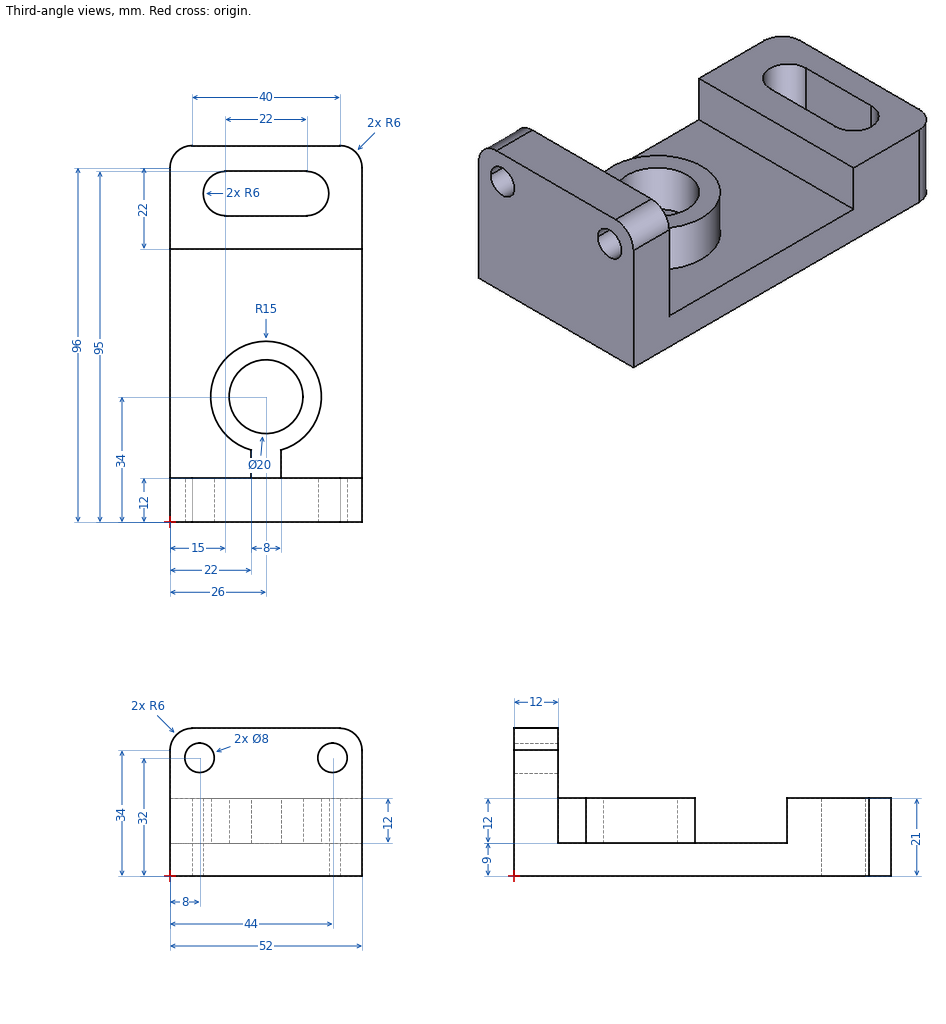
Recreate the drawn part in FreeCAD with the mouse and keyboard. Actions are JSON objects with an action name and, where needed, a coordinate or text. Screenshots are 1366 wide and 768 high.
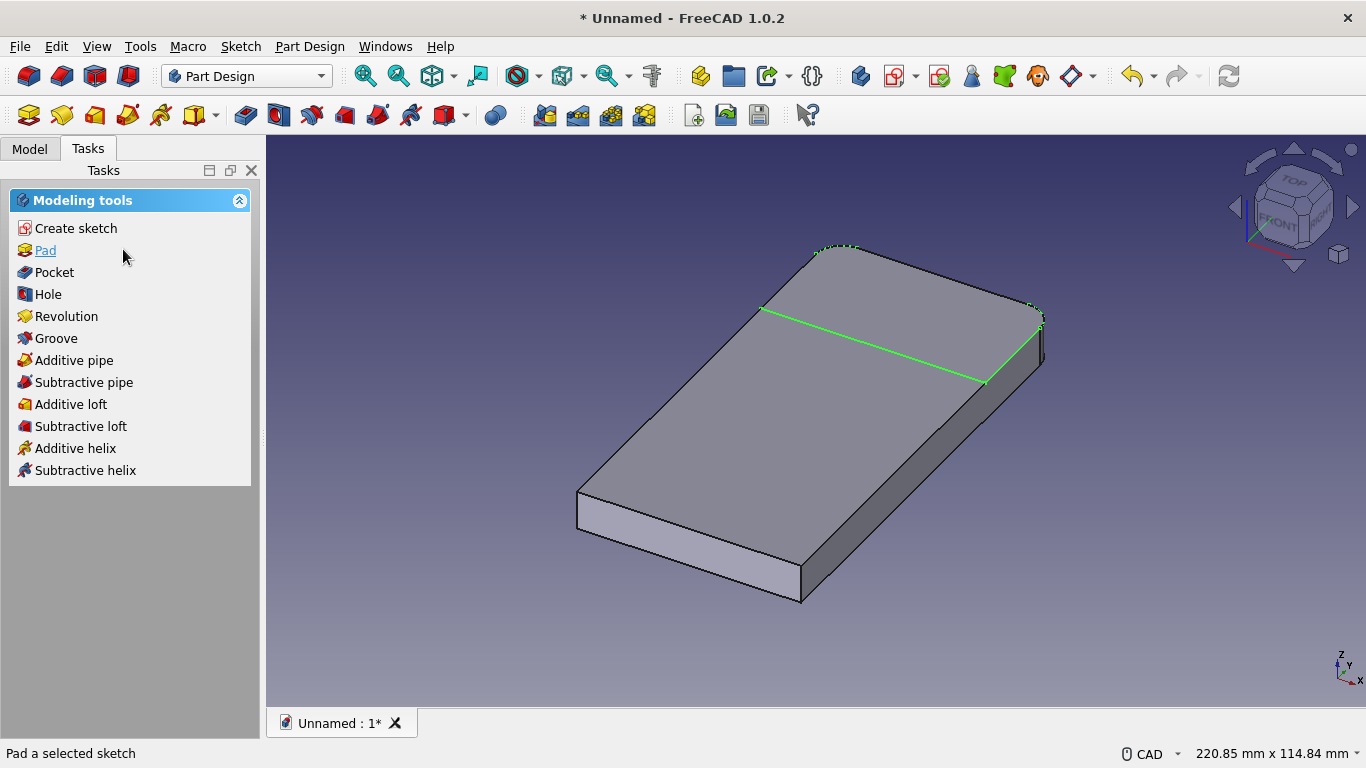
{"action": "left_click", "coordinate": [29, 116]}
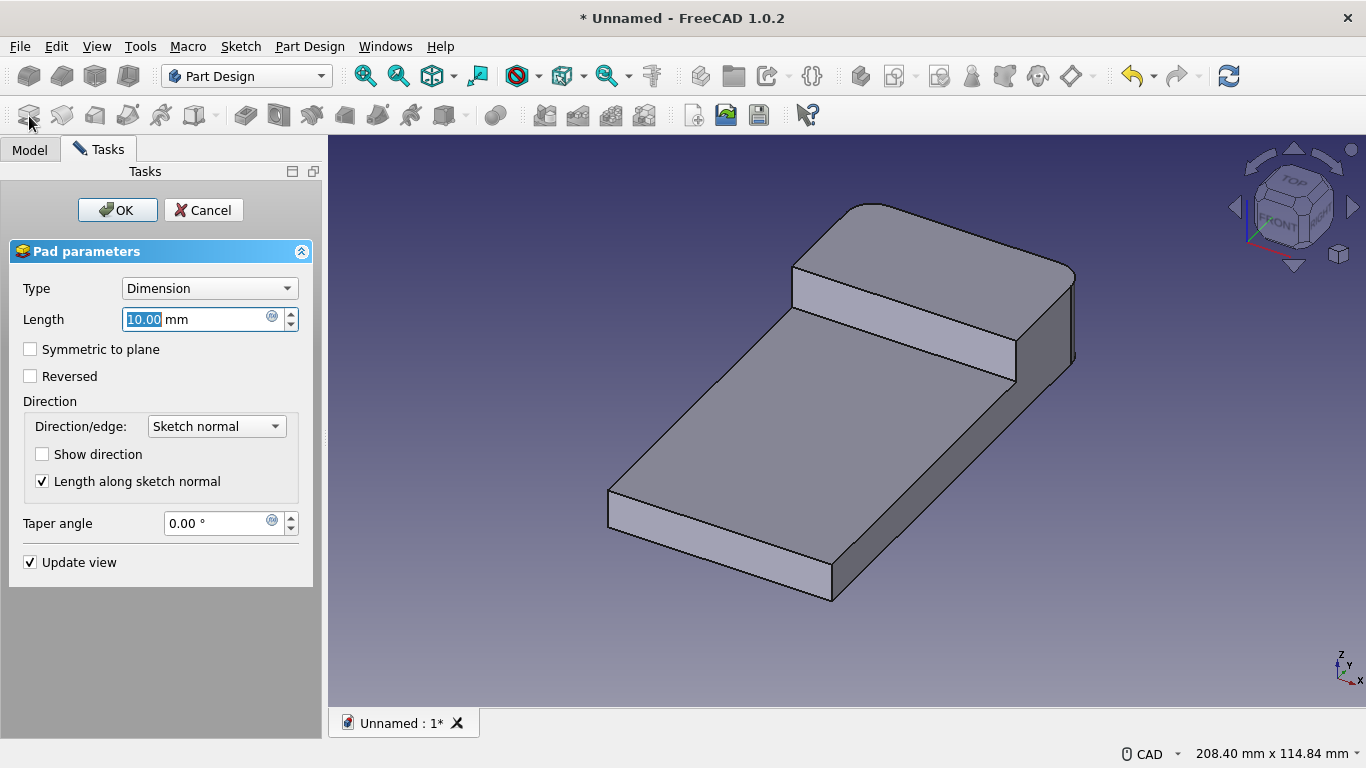
{"action": "type", "text": "12"}
{"action": "key", "text": "Tab"}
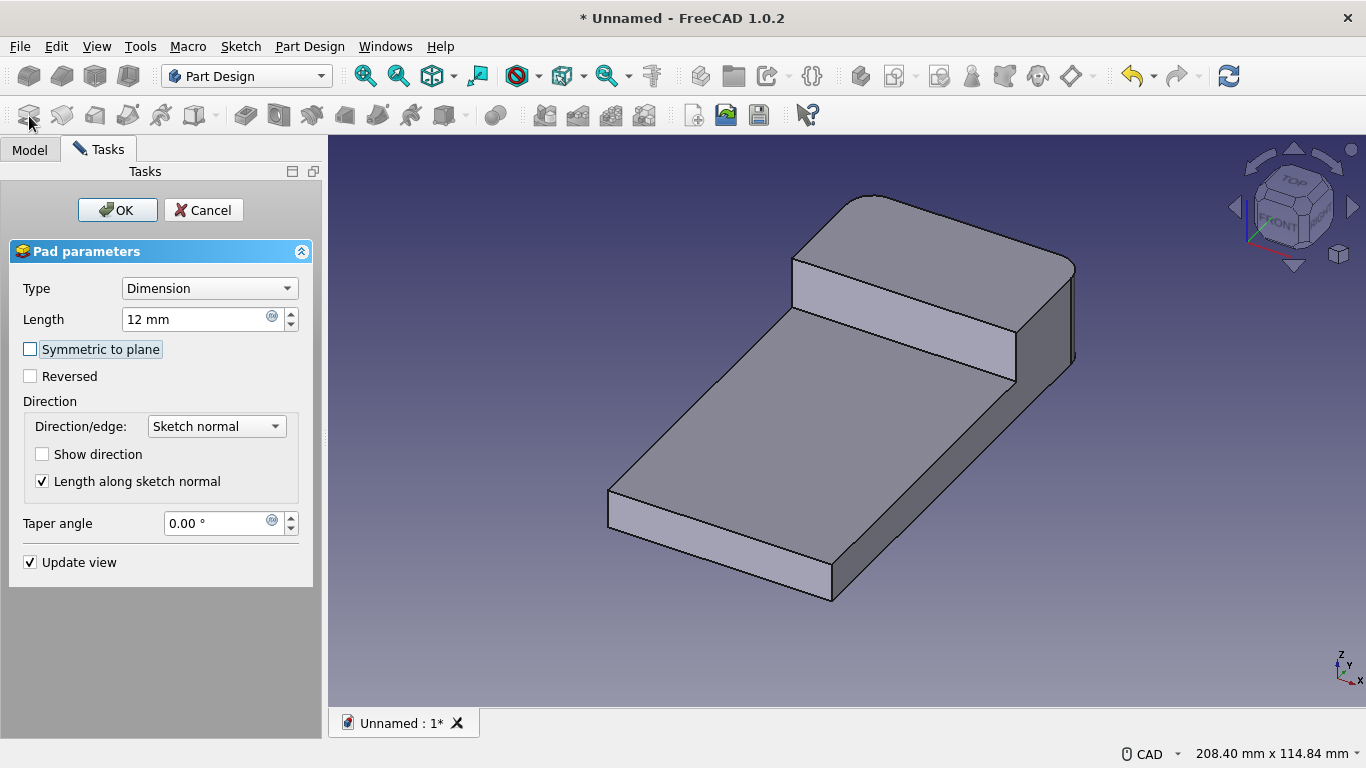
{"action": "left_click", "coordinate": [118, 210]}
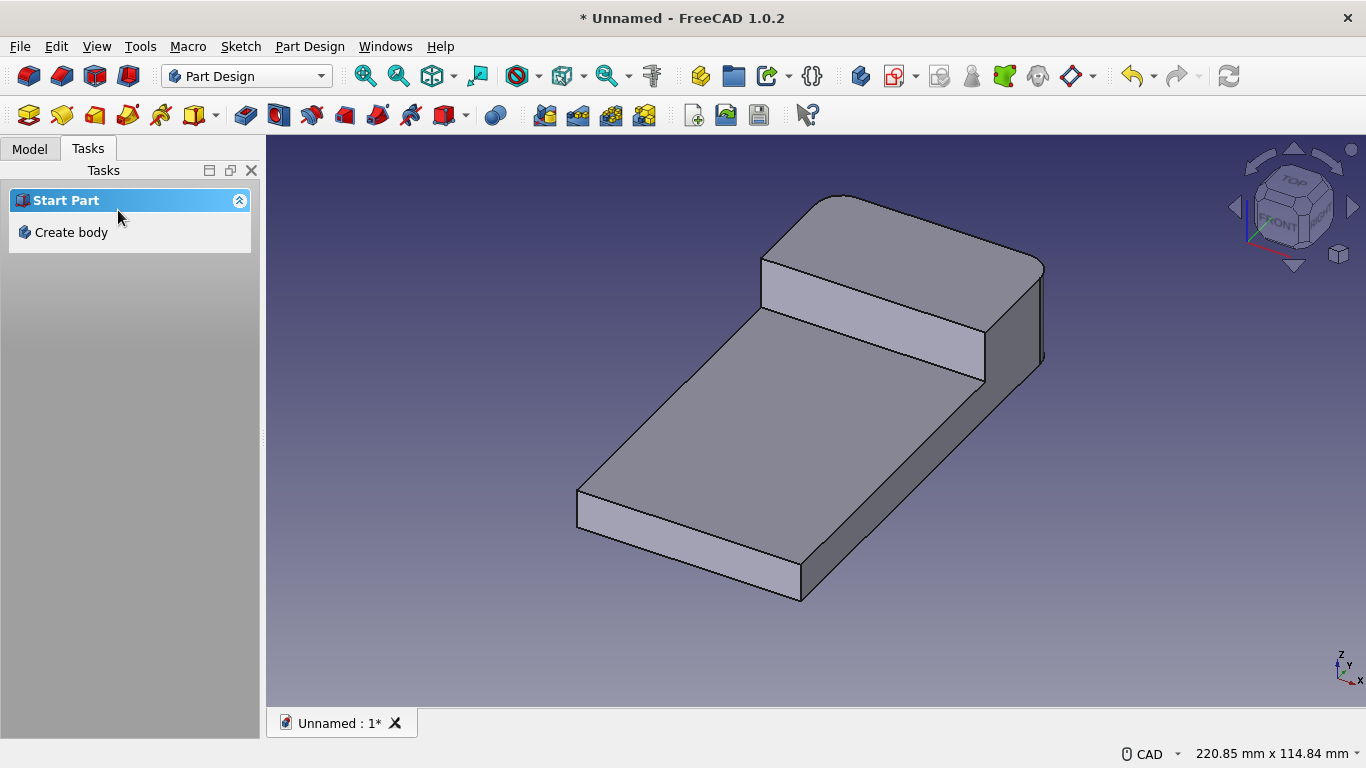
{"action": "left_click", "coordinate": [940, 271]}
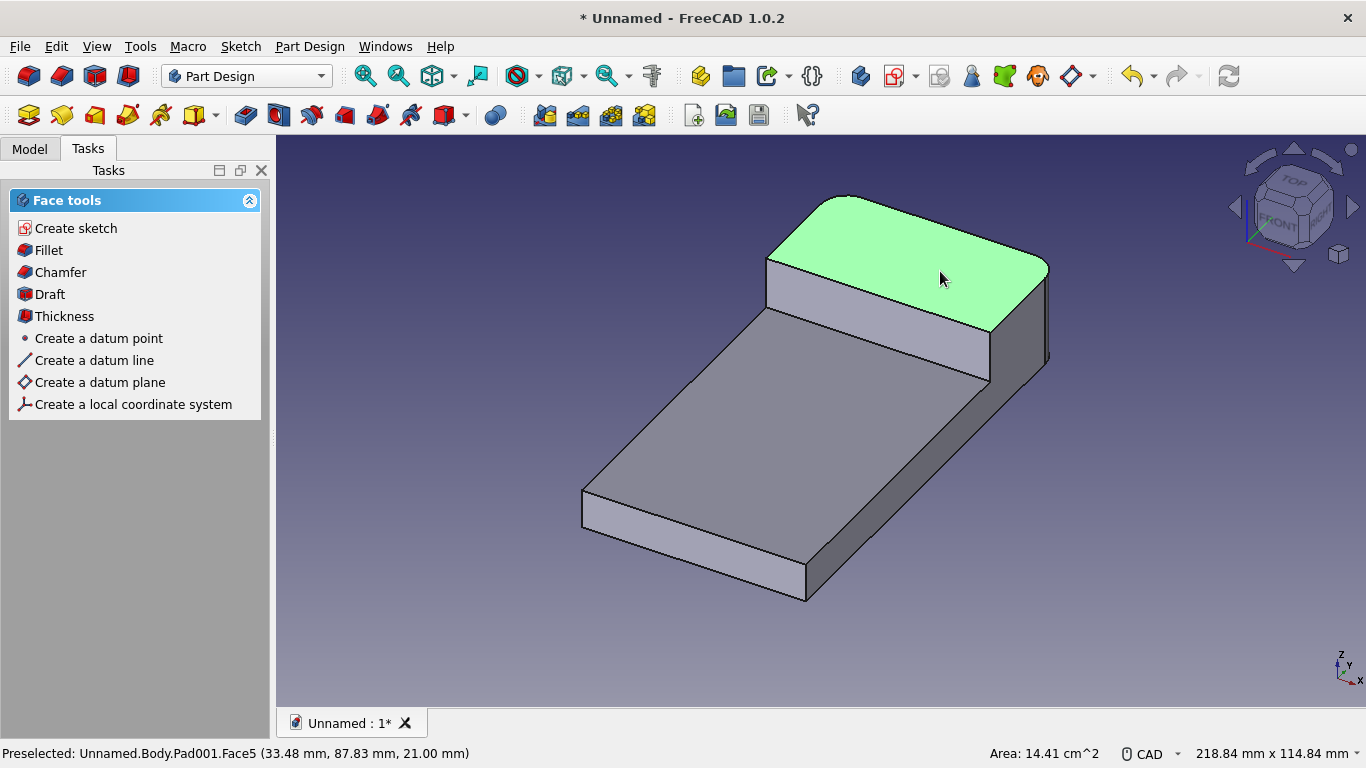
{"action": "left_click", "coordinate": [894, 76]}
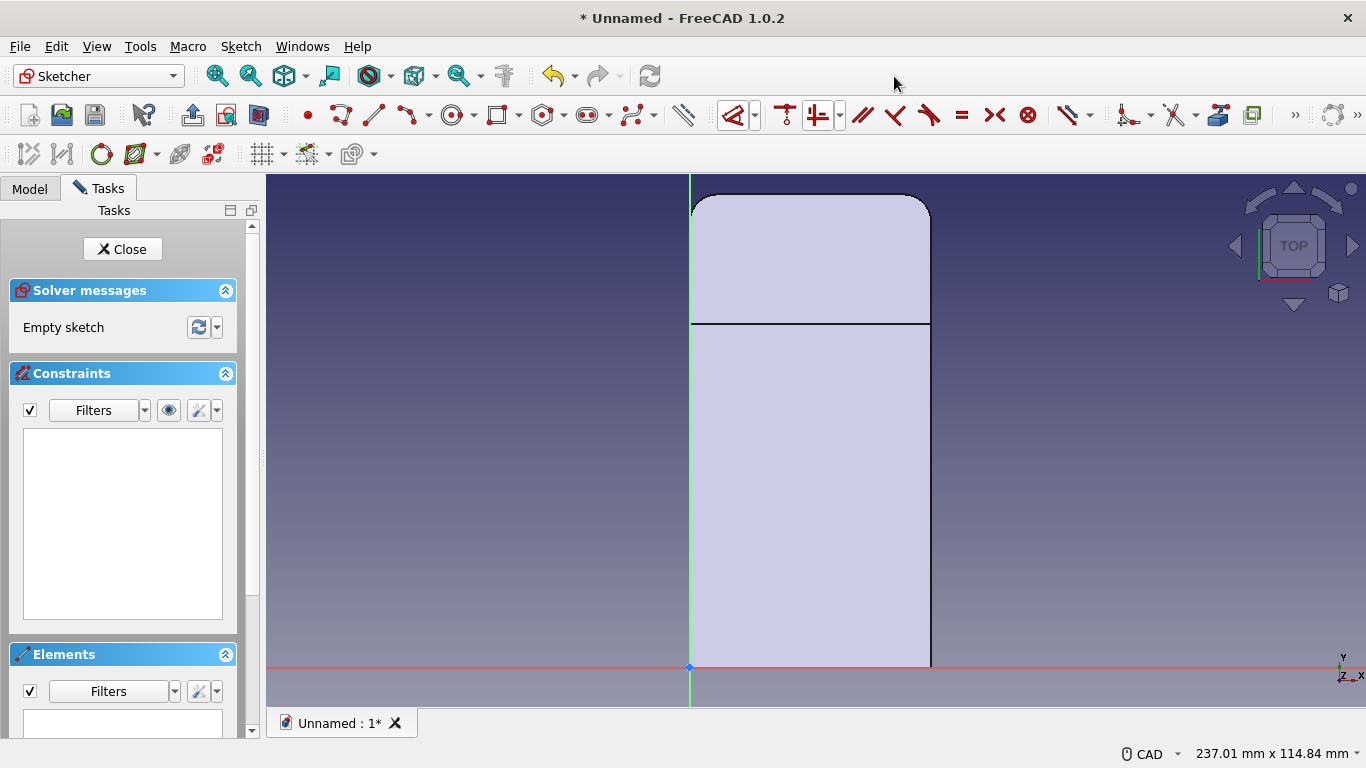
{"action": "scroll", "coordinate": [831, 202], "scroll_direction": "up", "scroll_amount": 7}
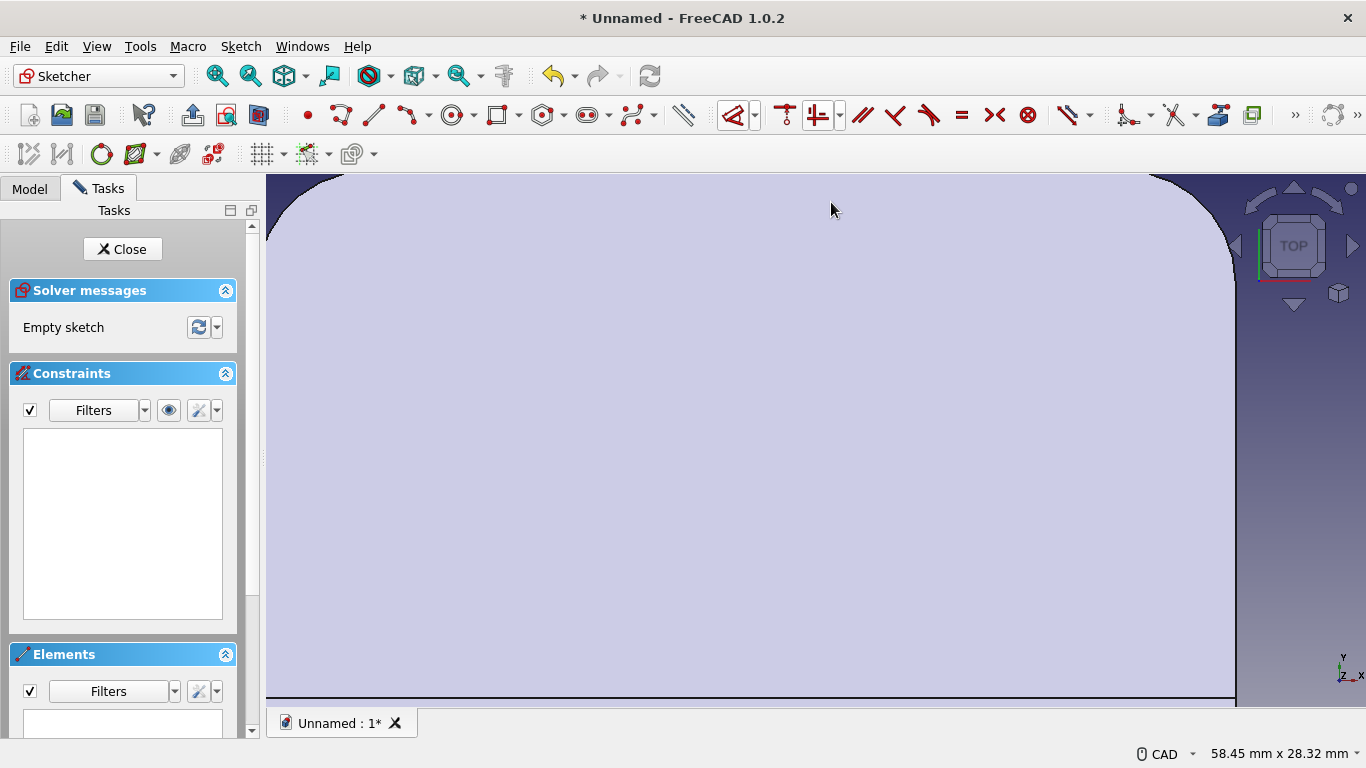
{"action": "left_click", "coordinate": [586, 116]}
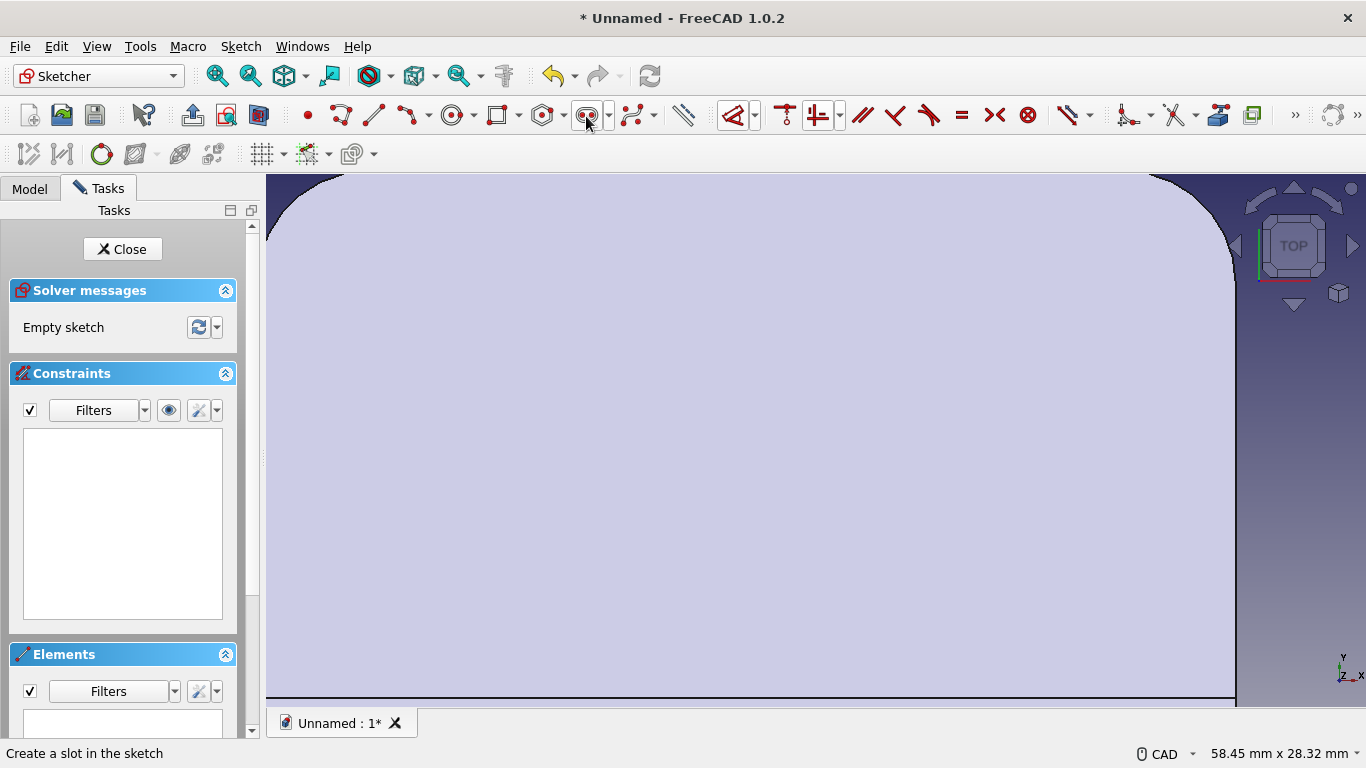
{"action": "left_click", "coordinate": [539, 415]}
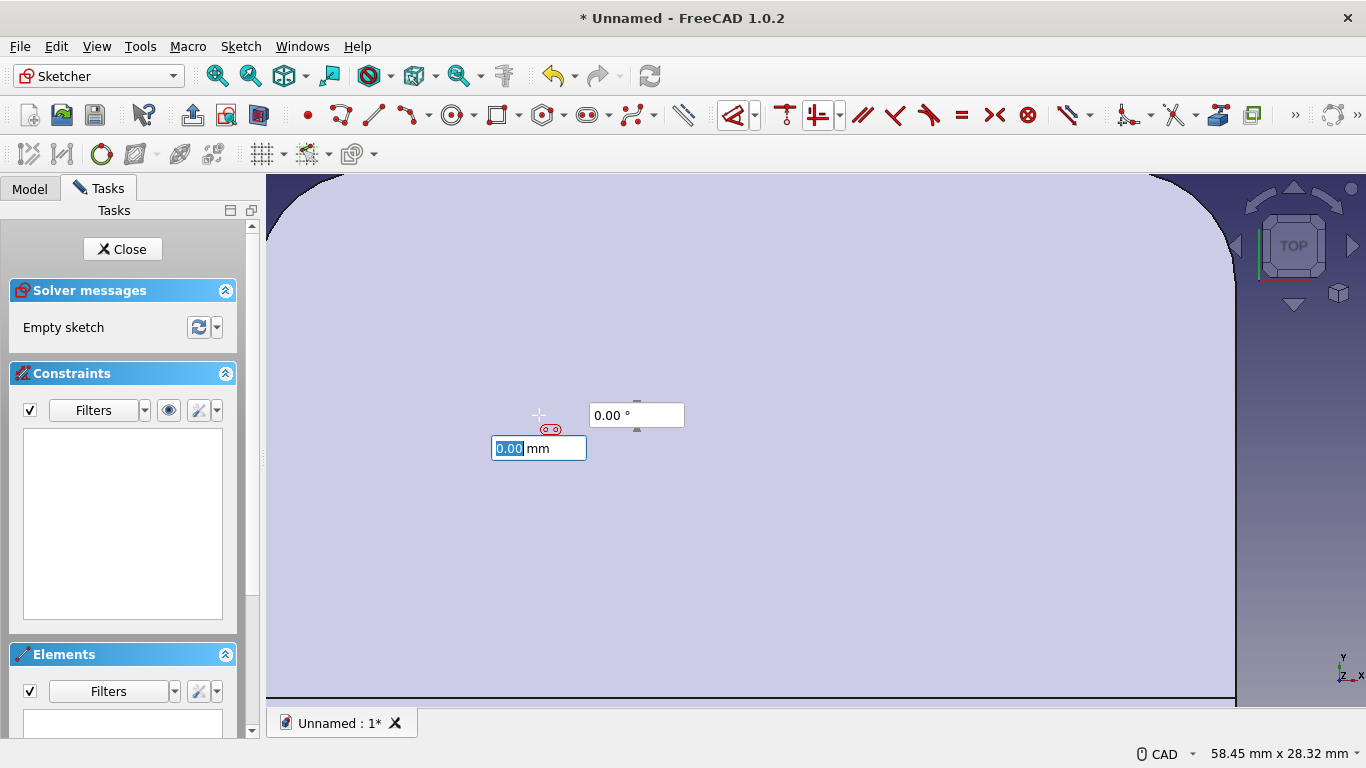
{"action": "left_click", "coordinate": [953, 415]}